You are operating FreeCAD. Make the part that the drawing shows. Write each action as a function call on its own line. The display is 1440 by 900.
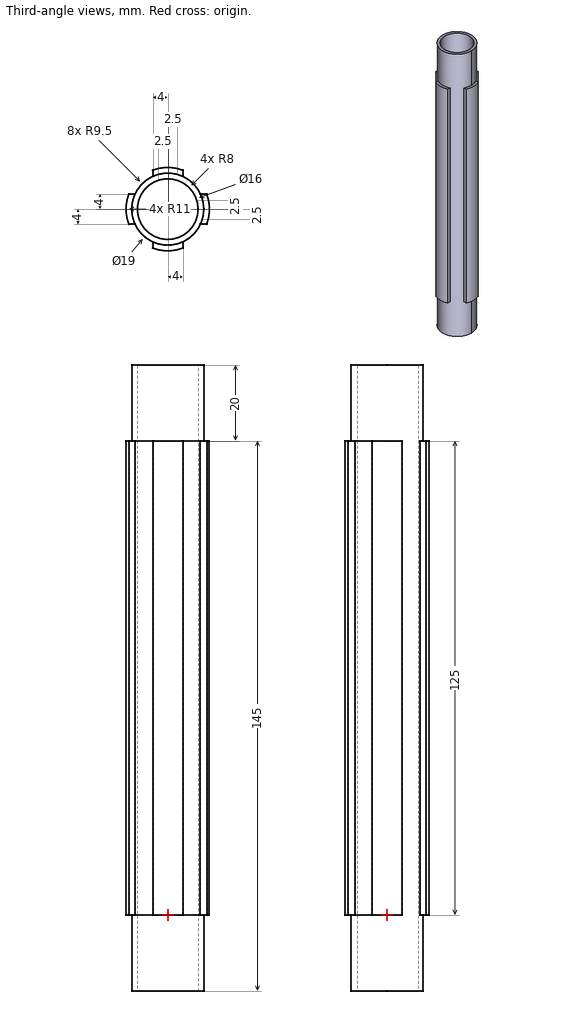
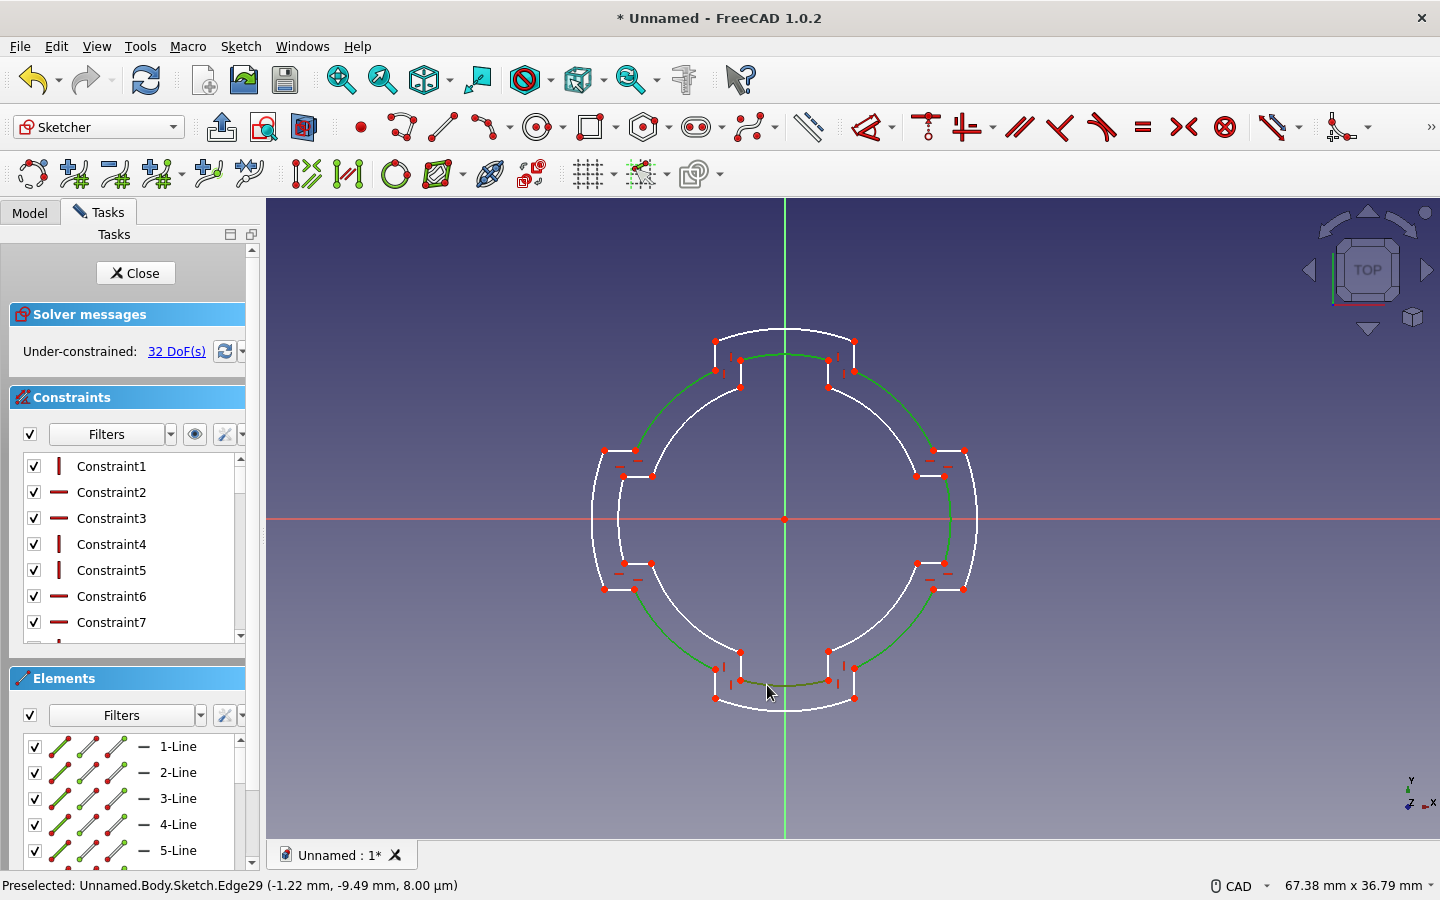
click(619, 503)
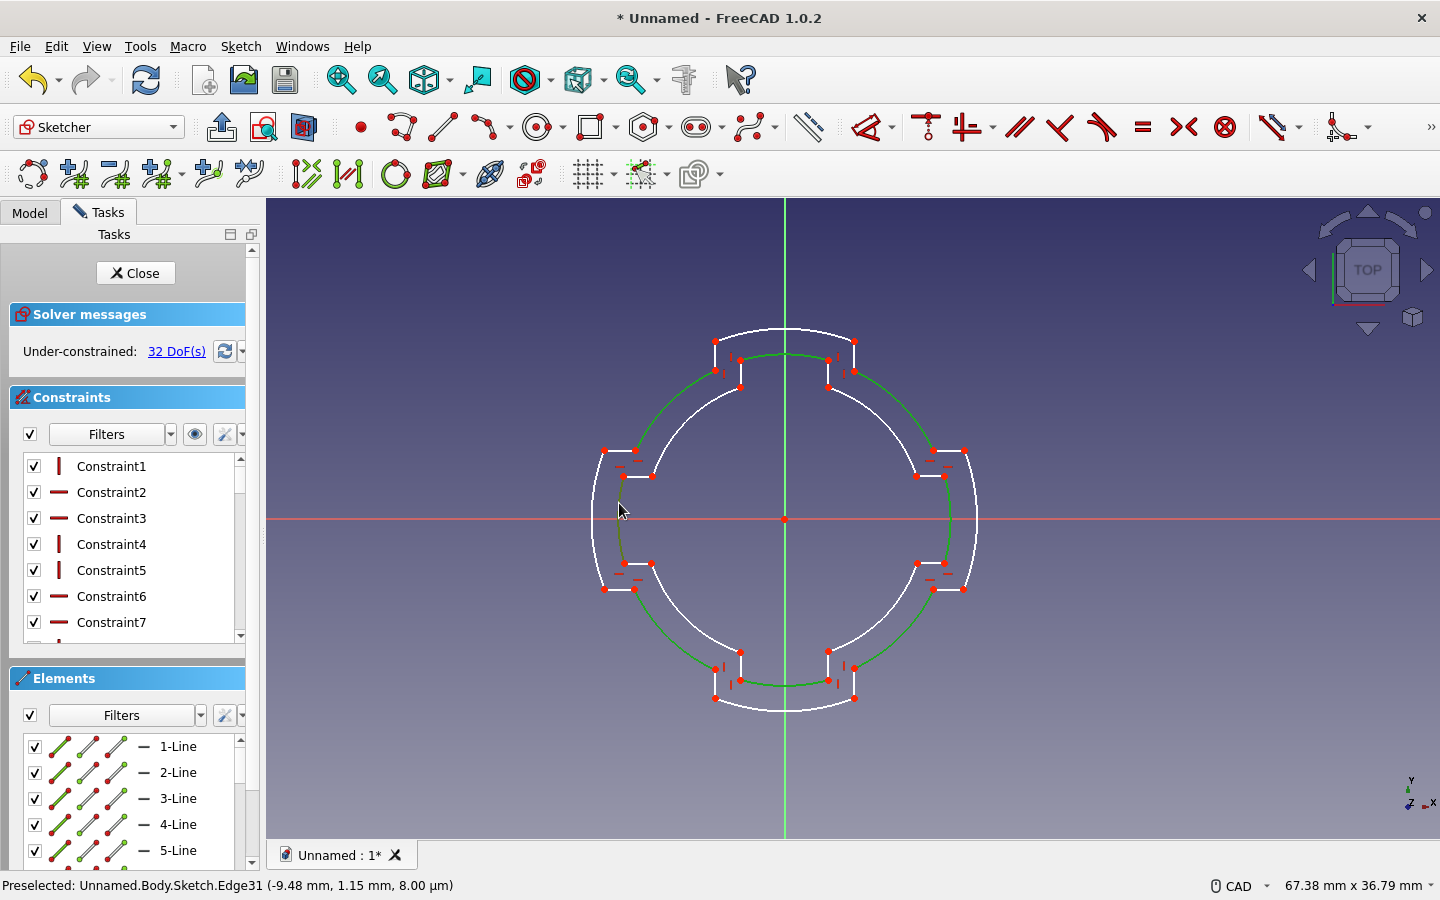
click(1143, 128)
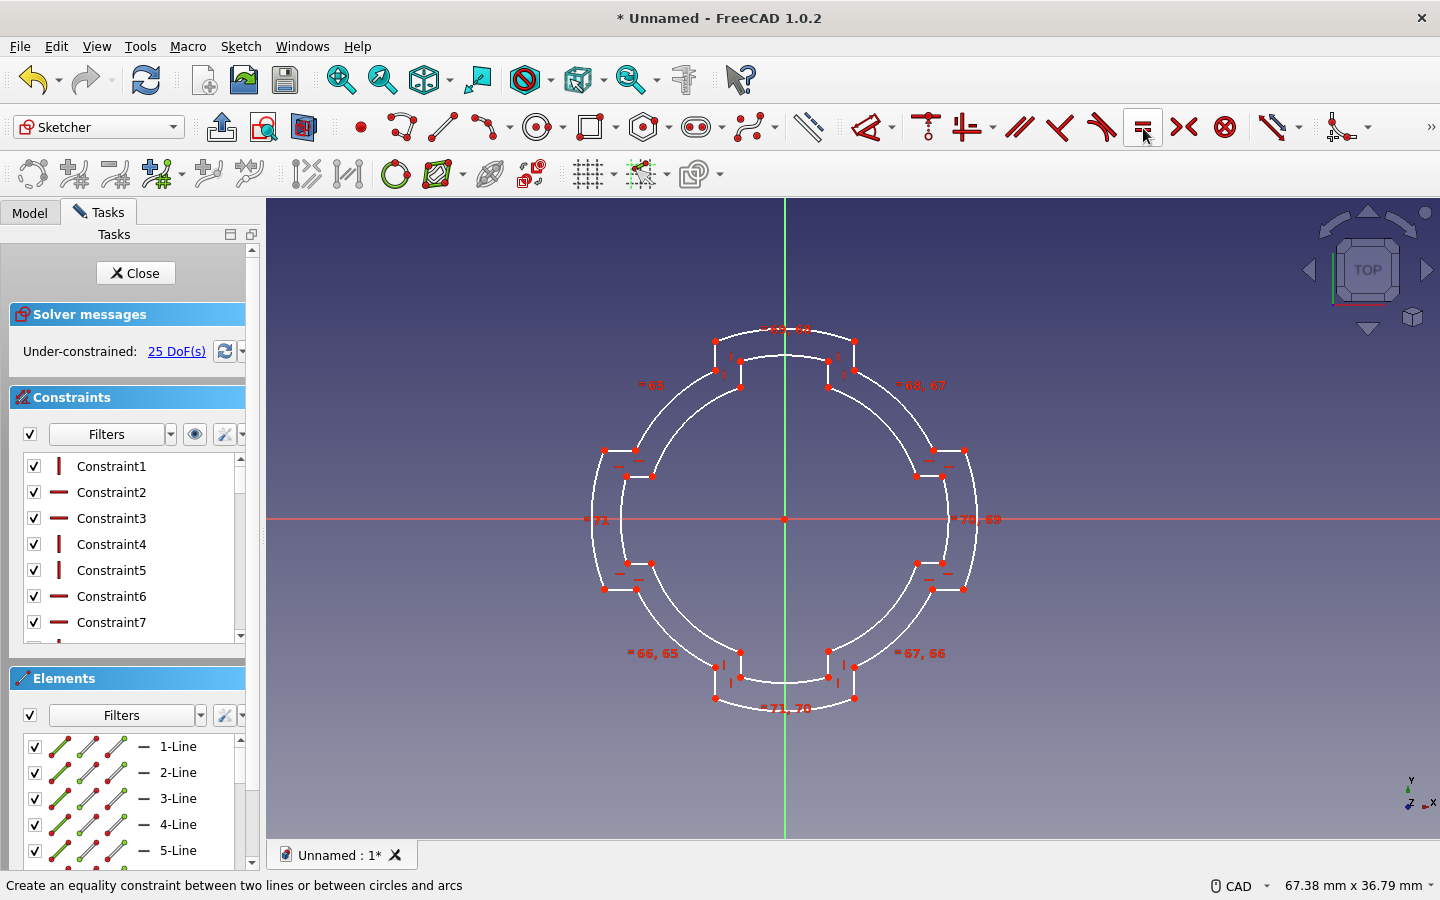
click(593, 492)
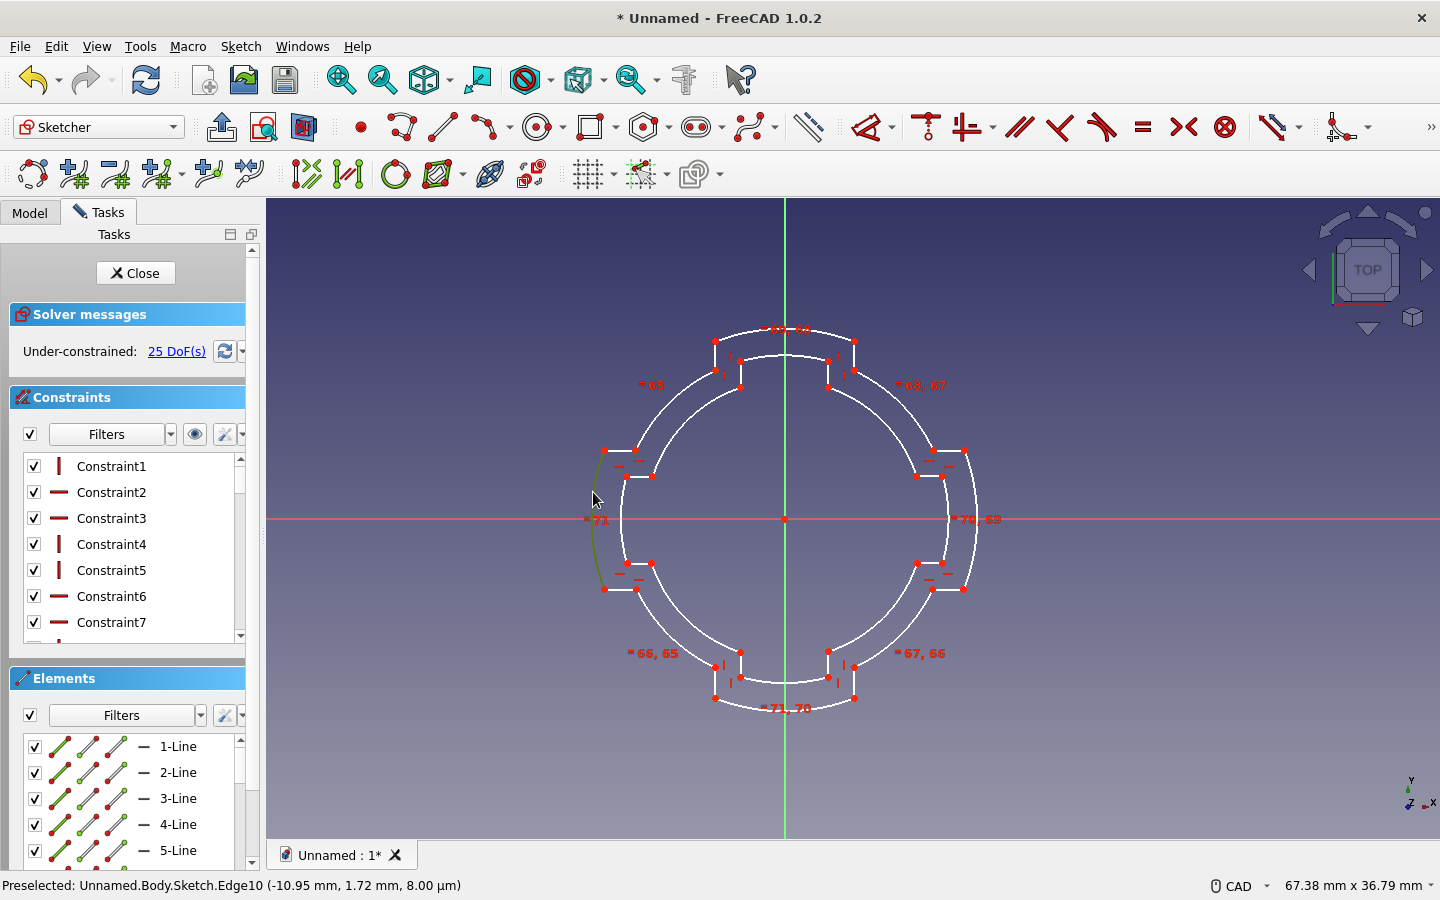
click(757, 709)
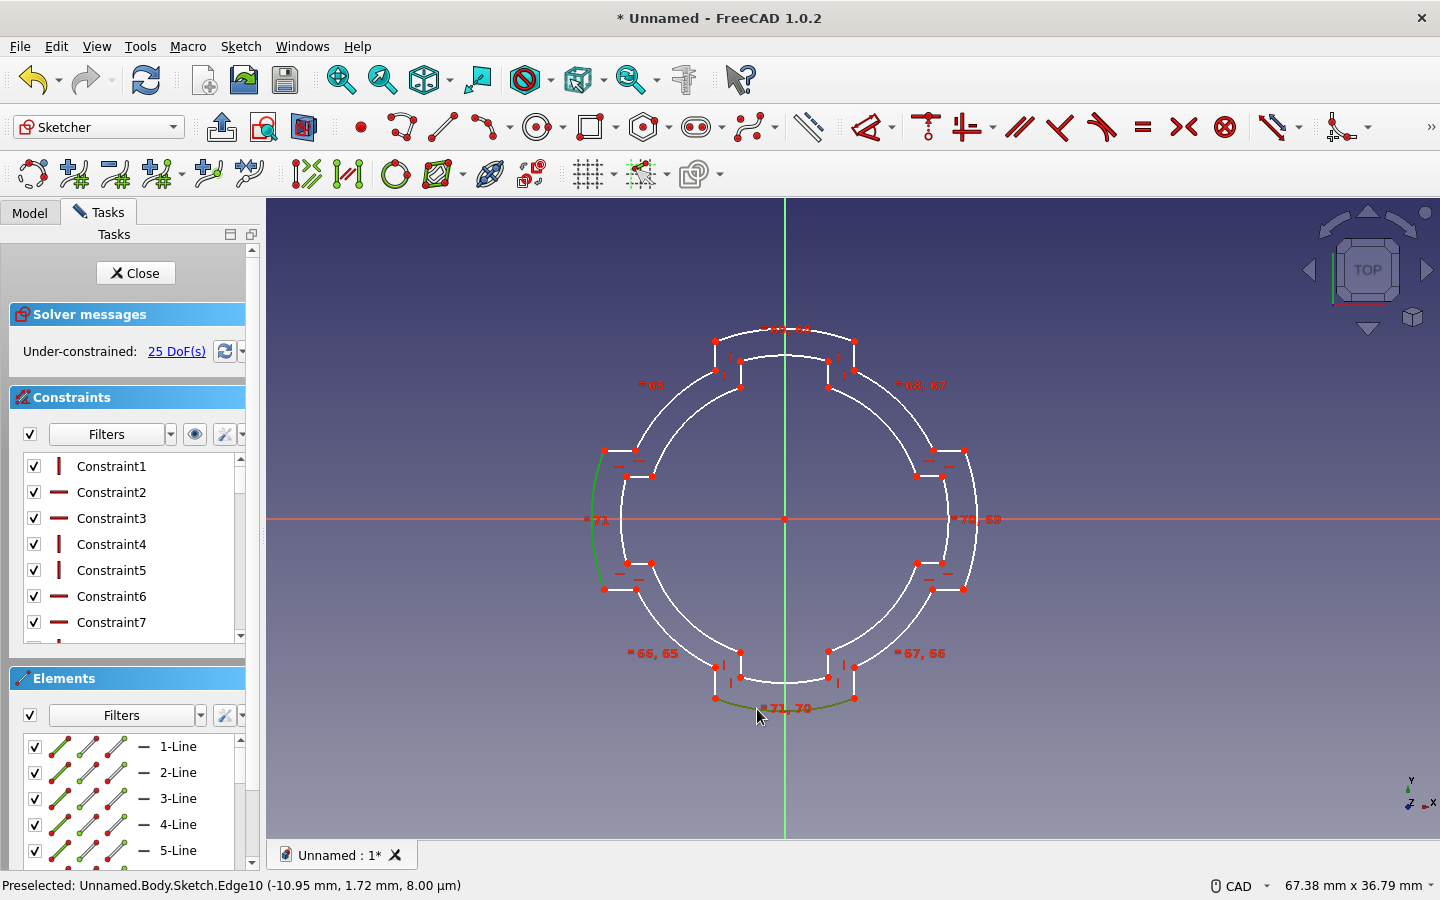
click(975, 549)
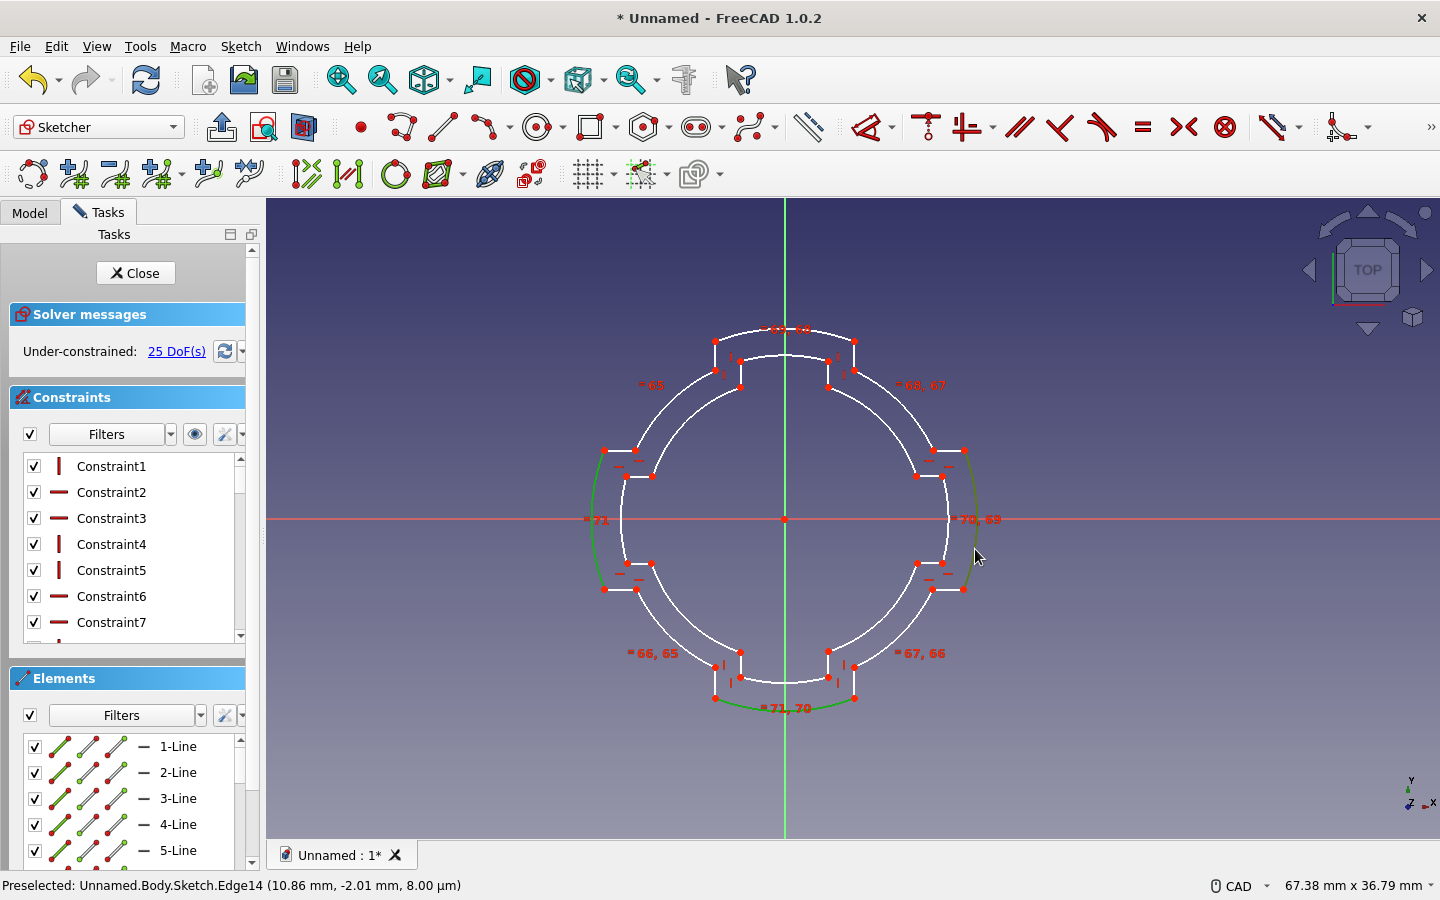
click(813, 331)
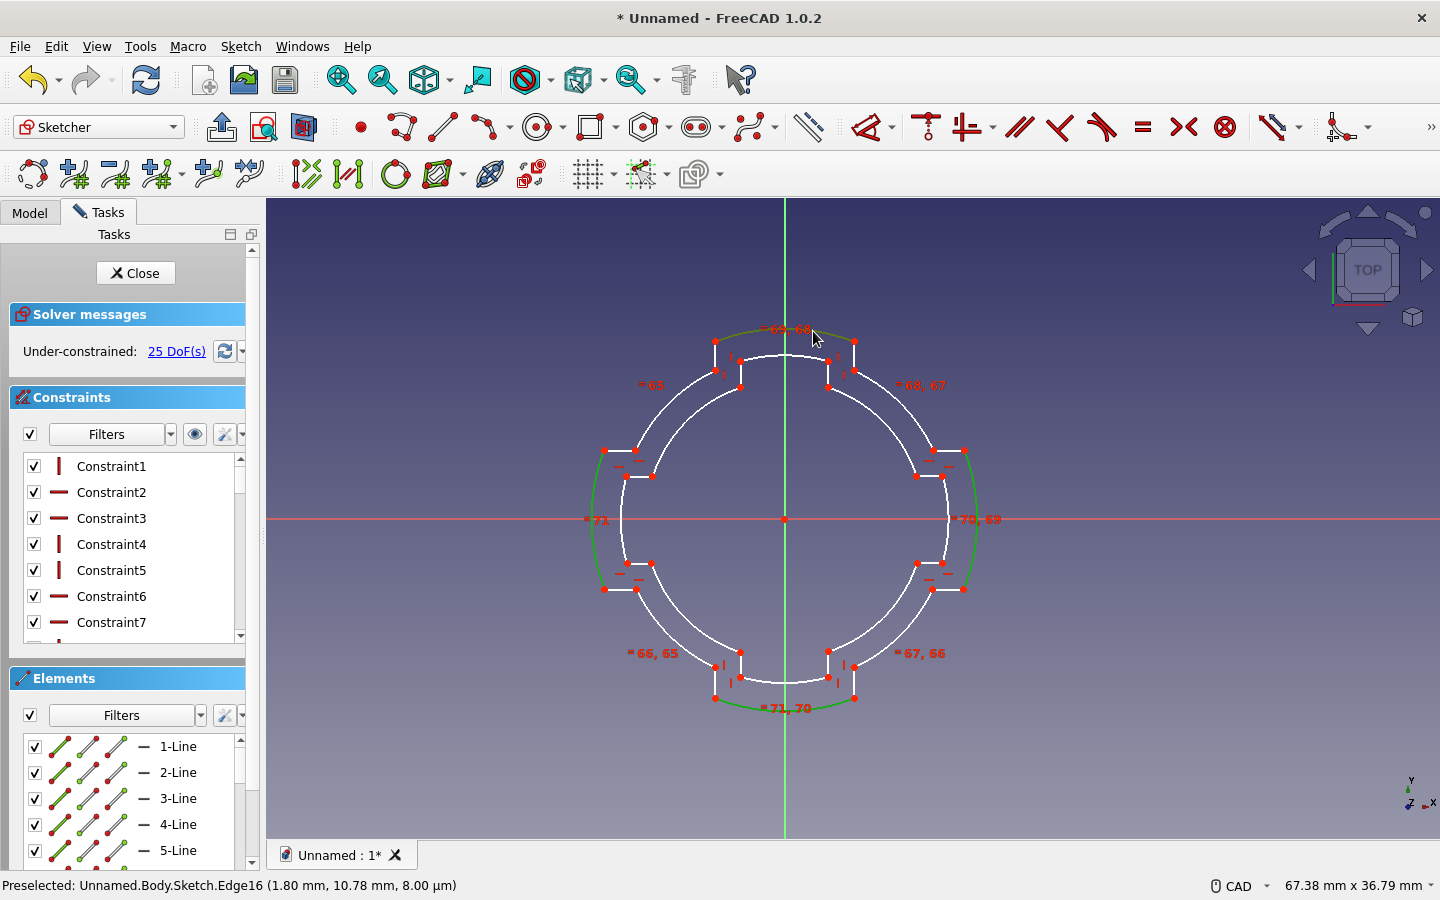
click(1143, 128)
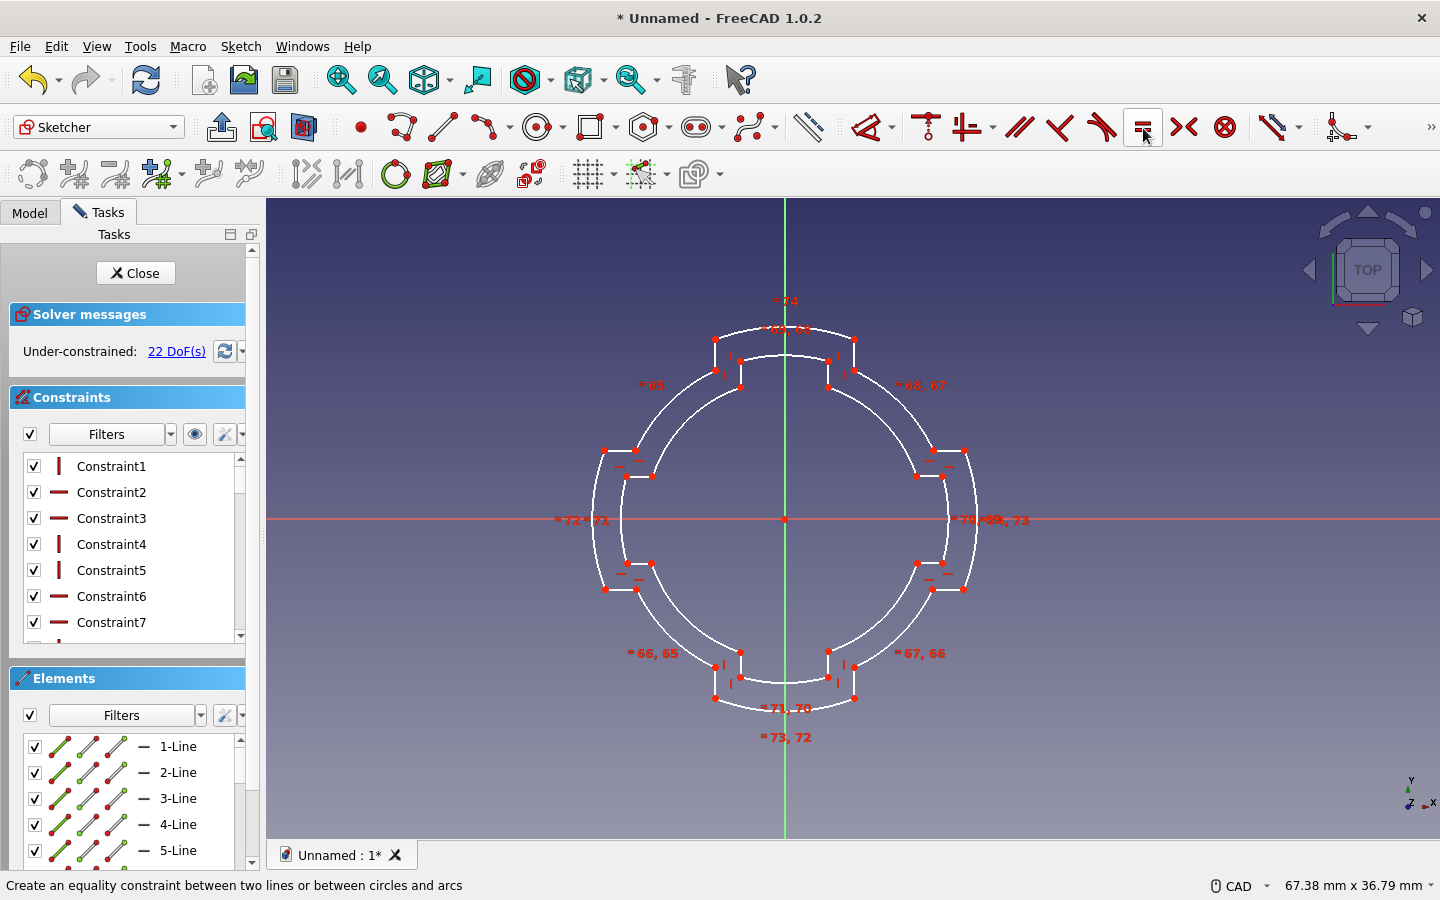
click(899, 441)